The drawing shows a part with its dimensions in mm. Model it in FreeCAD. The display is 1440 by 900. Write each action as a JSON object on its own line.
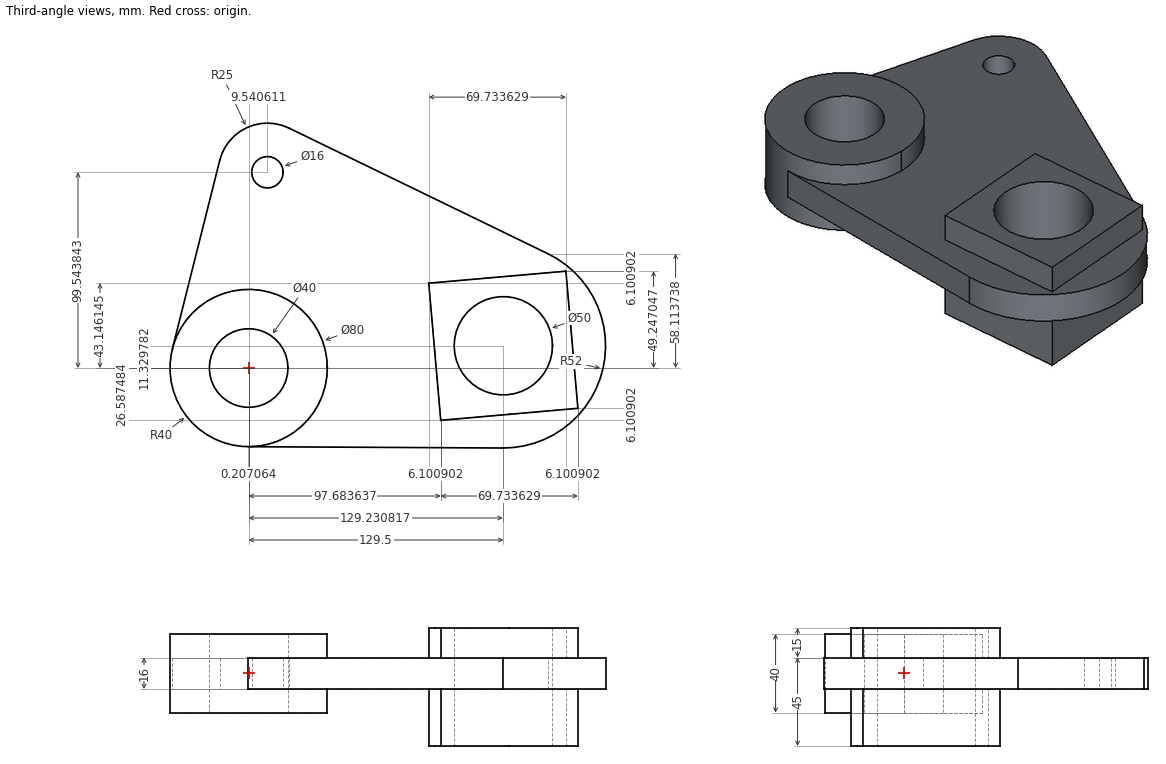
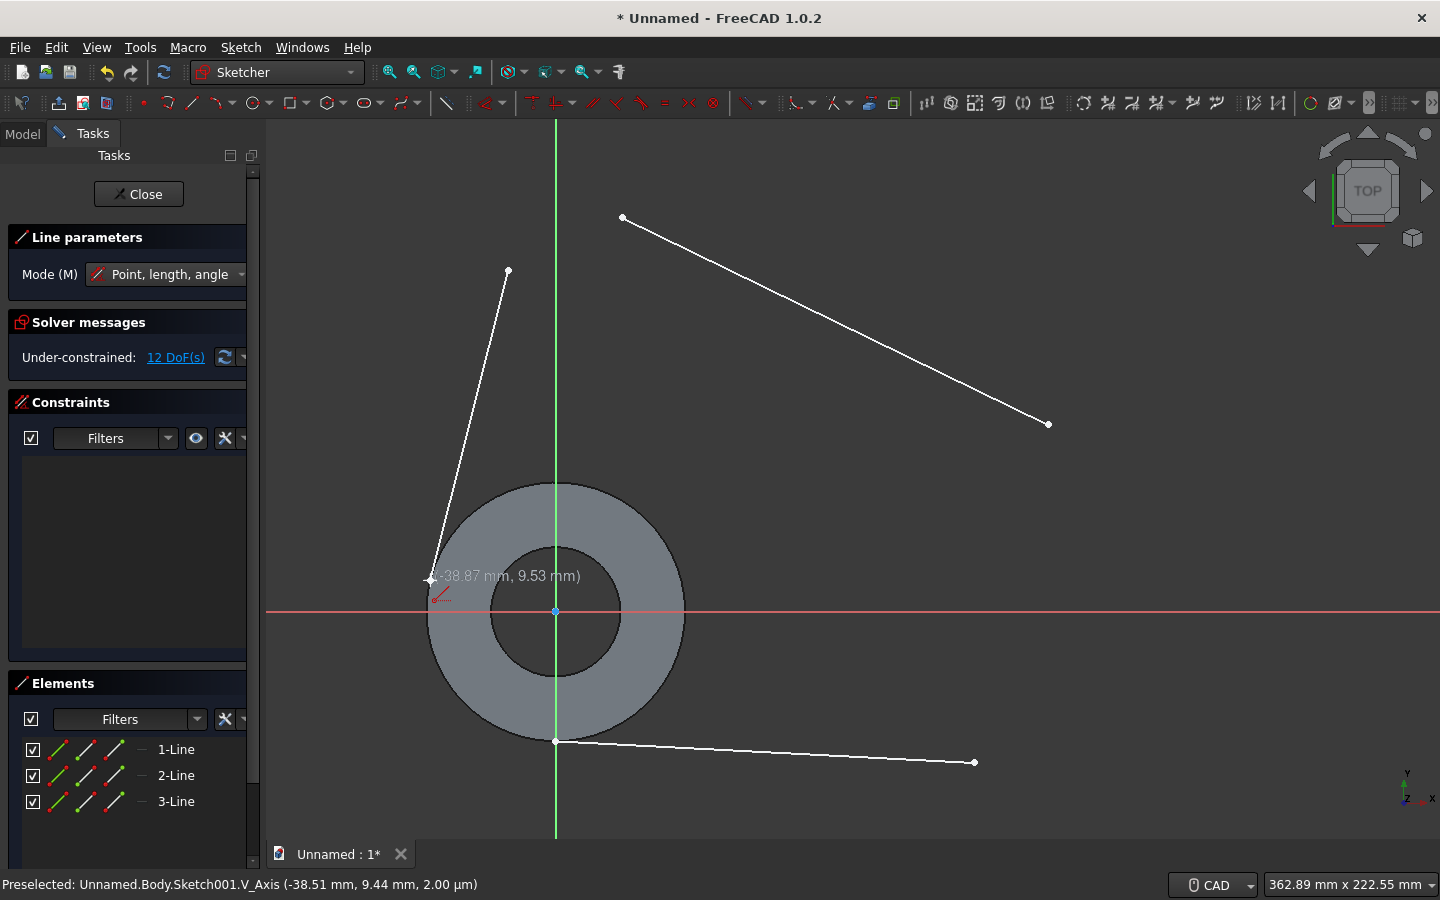
{"action": "key", "text": "g 3 a"}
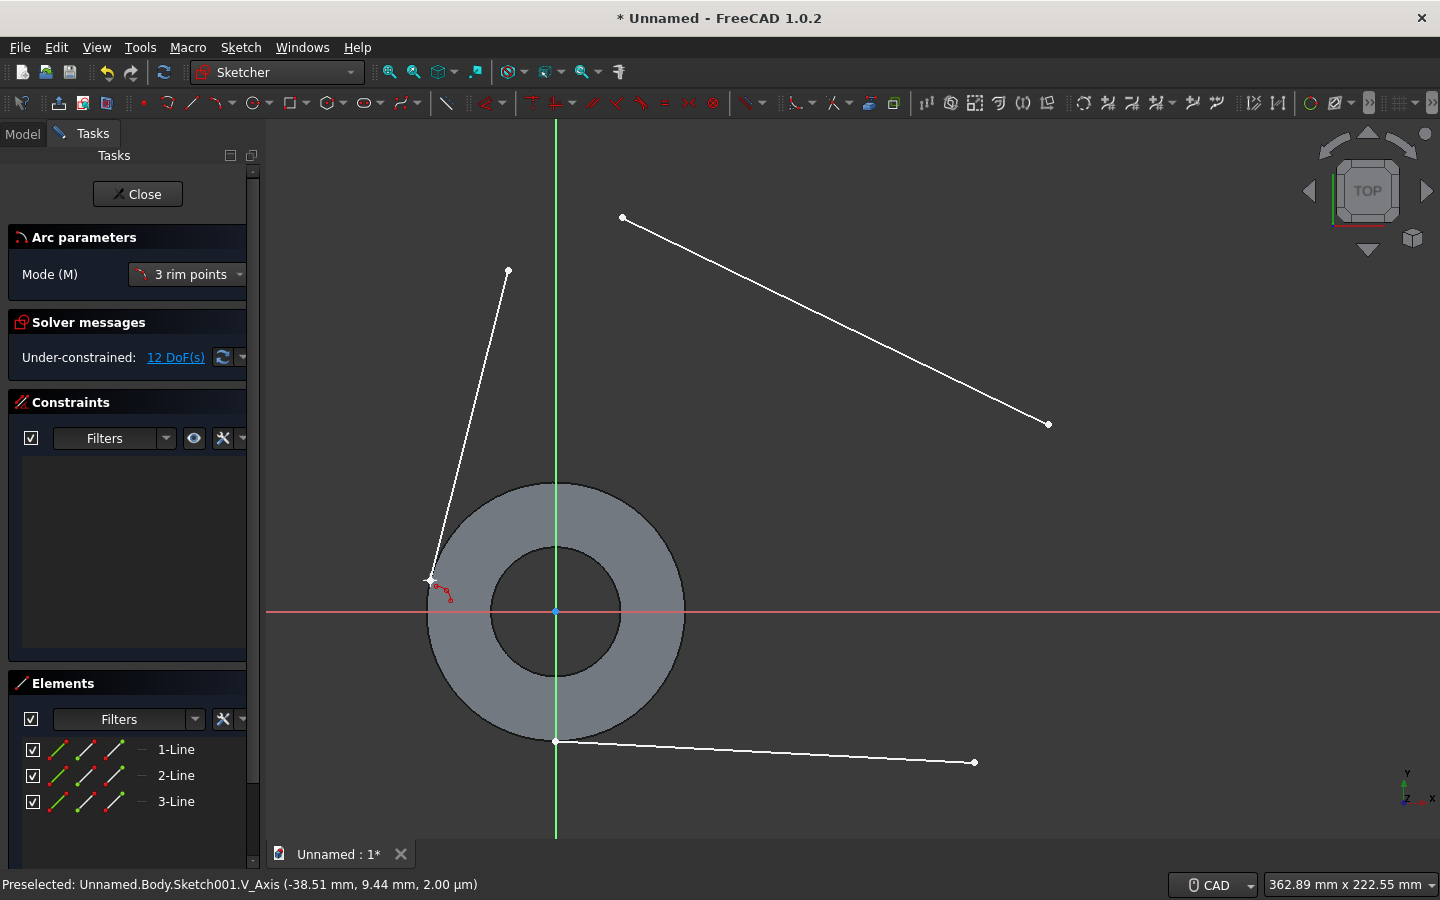
{"action": "left_click", "coordinate": [974, 763]}
{"action": "left_click", "coordinate": [1048, 425]}
{"action": "left_click", "coordinate": [1123, 656]}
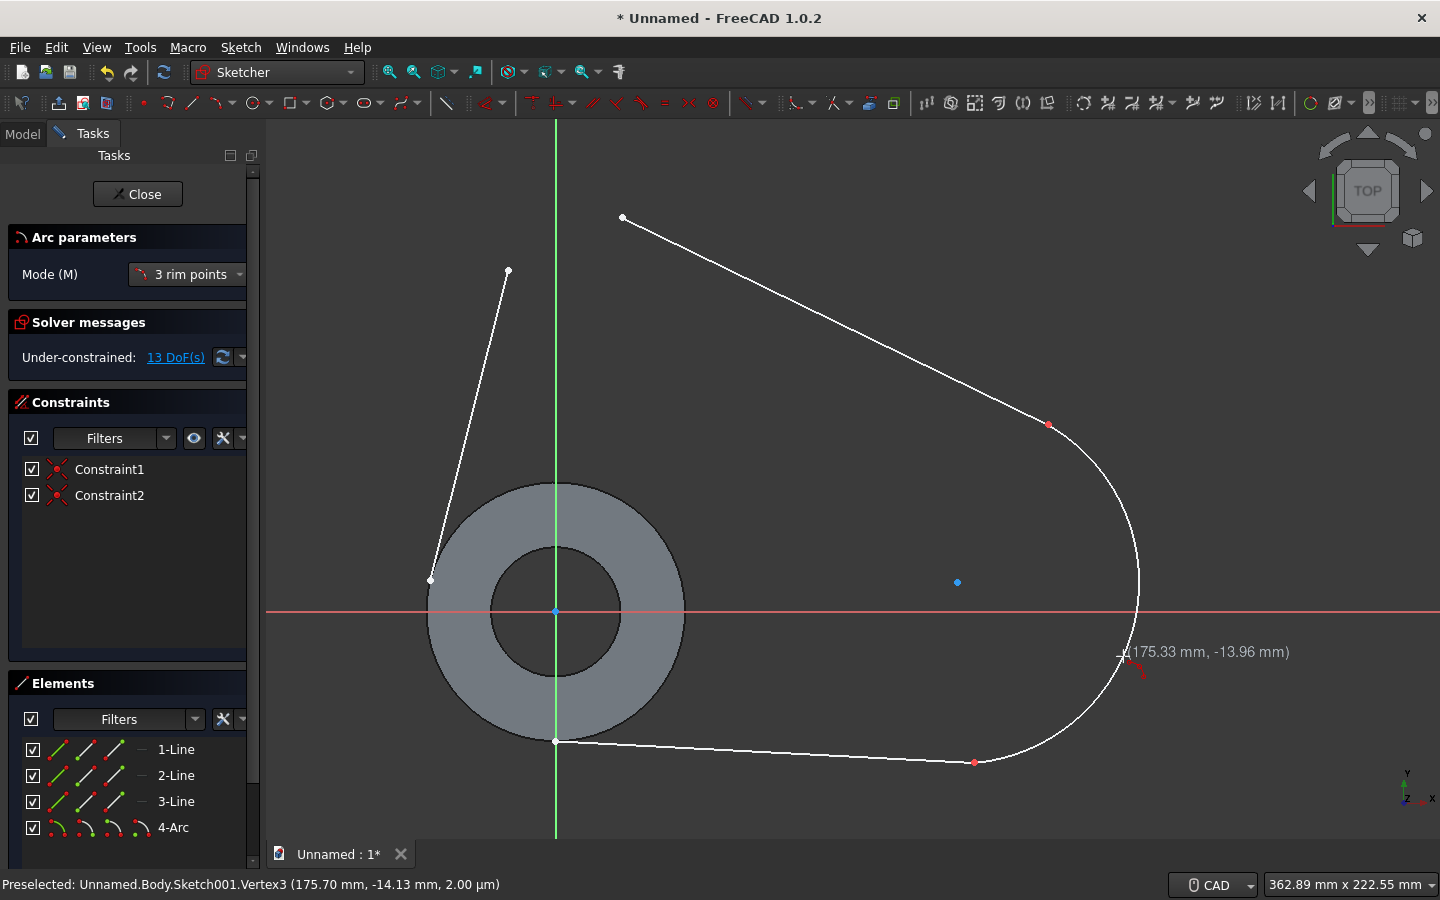
{"action": "left_click", "coordinate": [622, 218]}
{"action": "left_click", "coordinate": [508, 271]}
{"action": "left_click", "coordinate": [580, 209]}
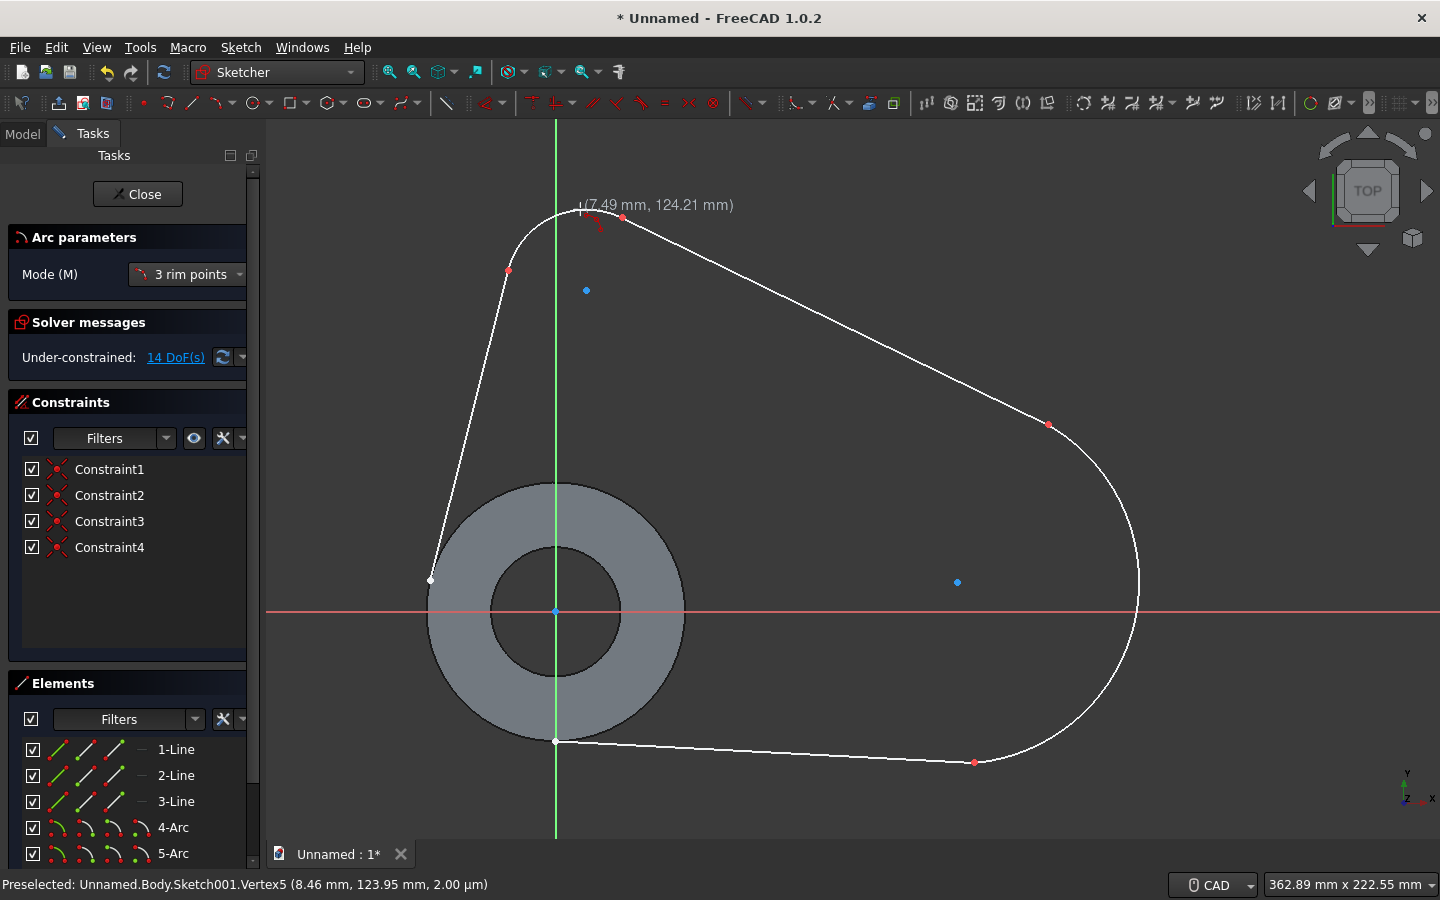
{"action": "left_click", "coordinate": [430, 581]}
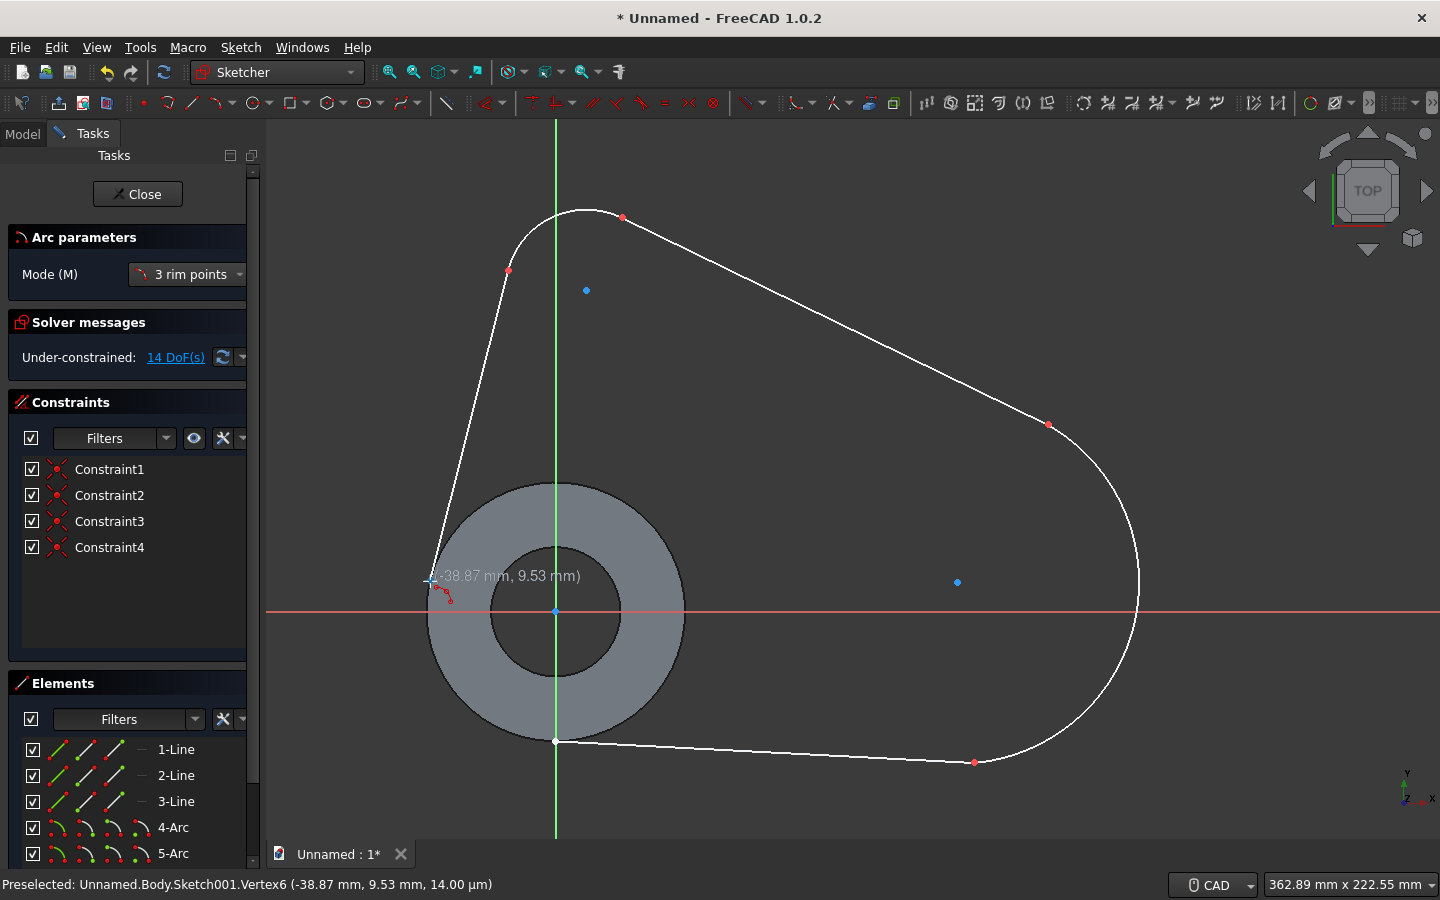
{"action": "scroll", "coordinate": [555, 741], "scroll_direction": "up", "scroll_amount": 16}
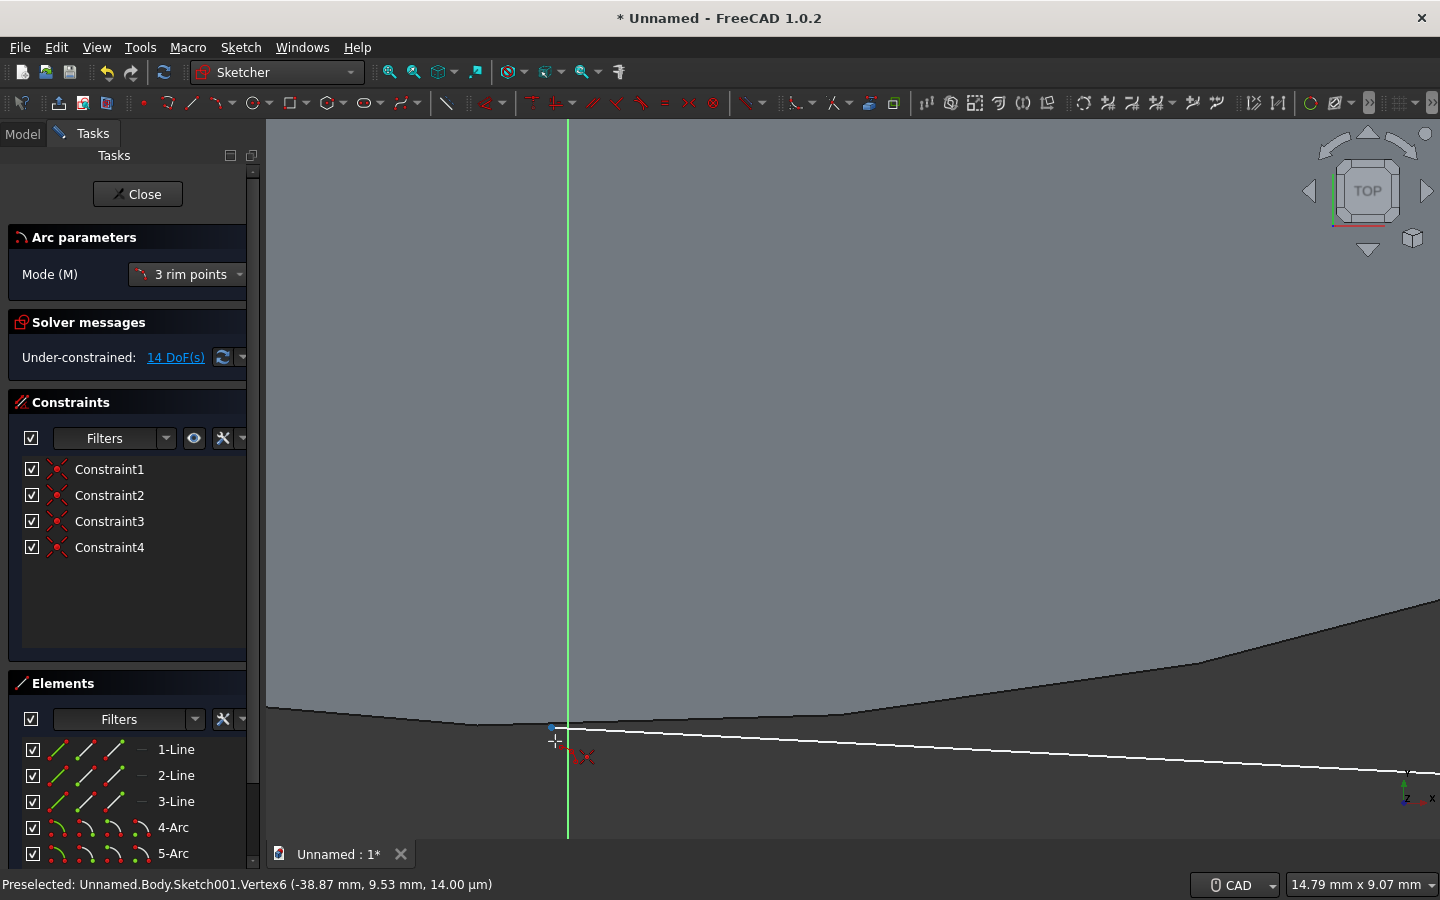
{"action": "left_click", "coordinate": [551, 728]}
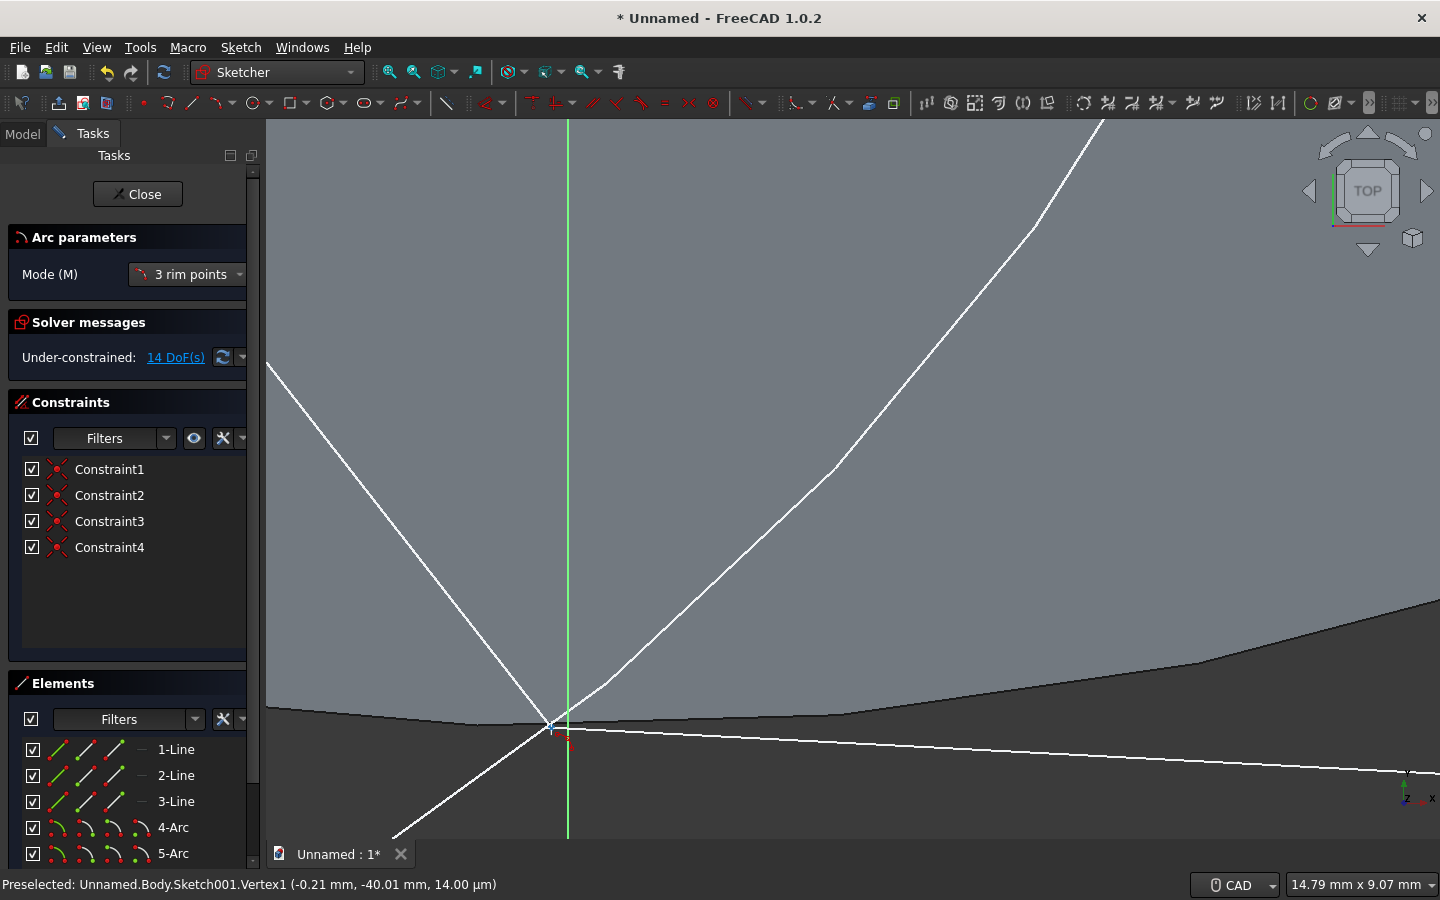
{"action": "scroll", "coordinate": [555, 741], "scroll_direction": "down", "scroll_amount": 16}